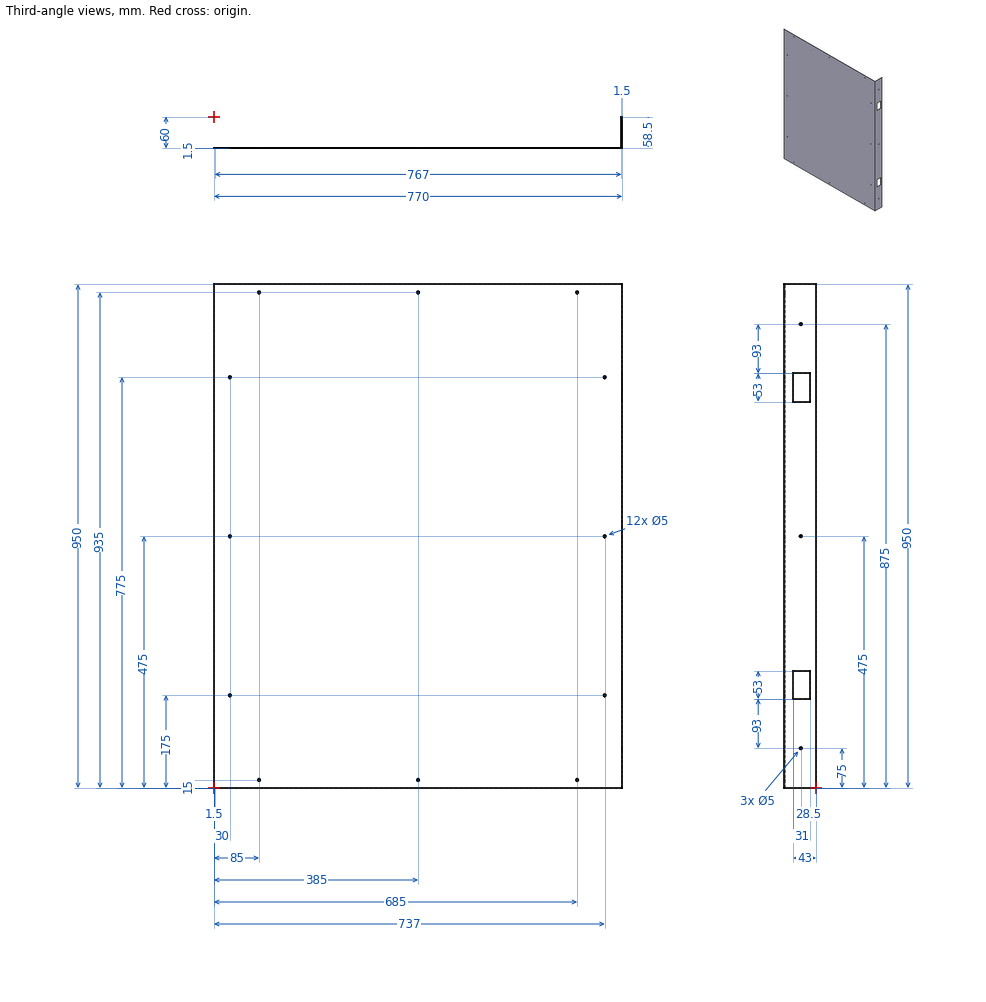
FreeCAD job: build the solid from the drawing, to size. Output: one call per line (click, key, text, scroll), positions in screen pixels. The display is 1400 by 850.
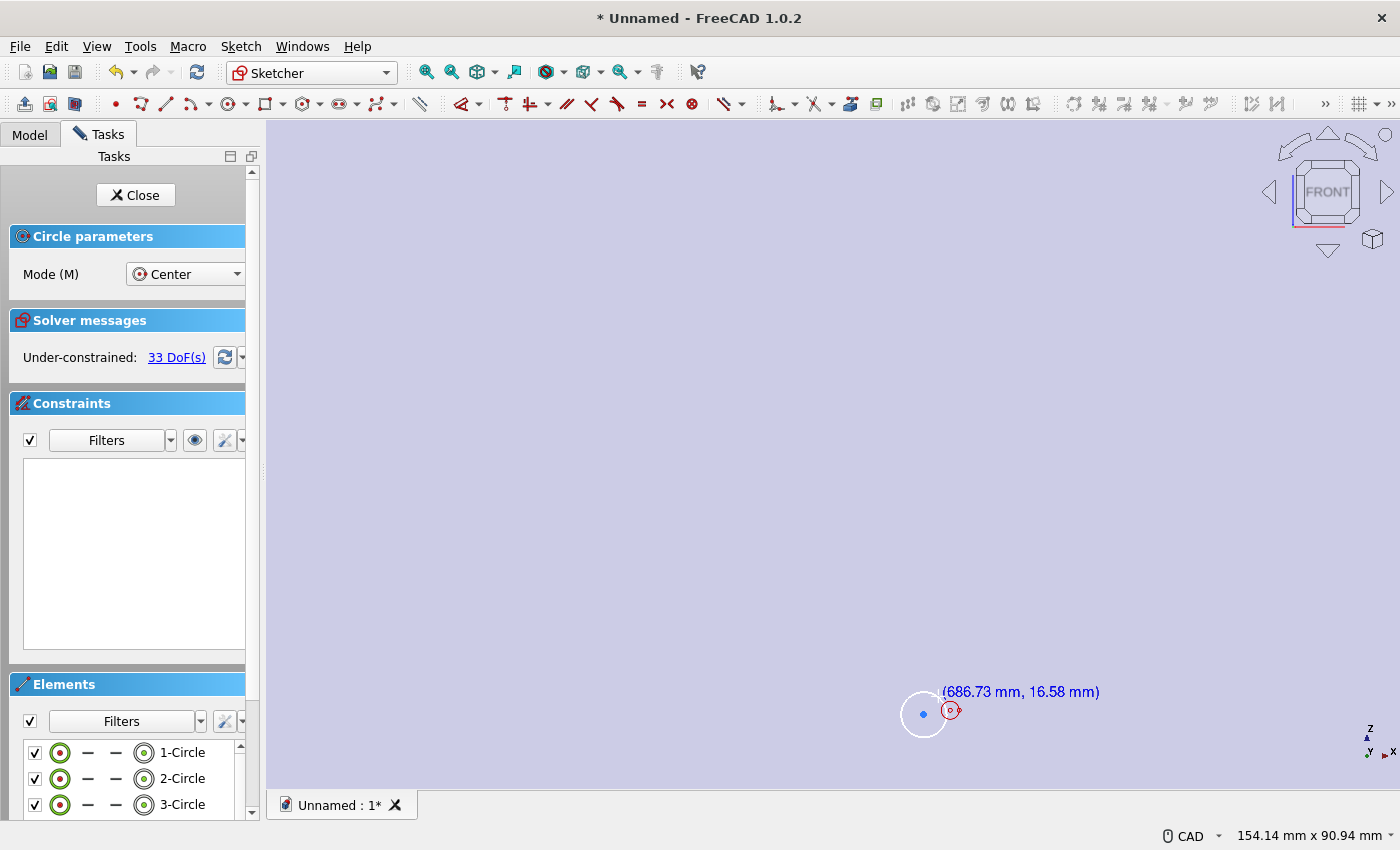
scroll(904, 654, down, 14)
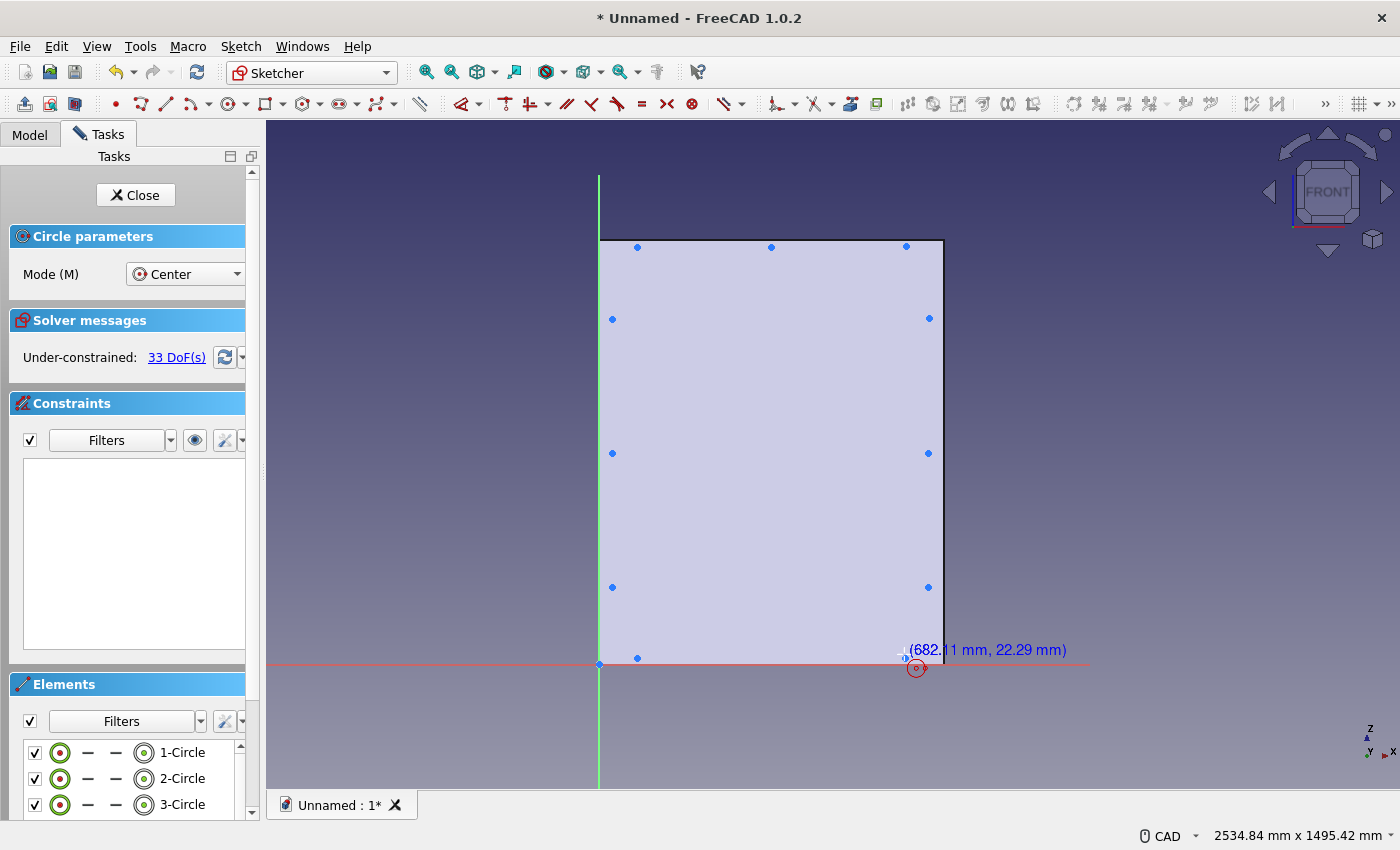
scroll(772, 658, up, 16)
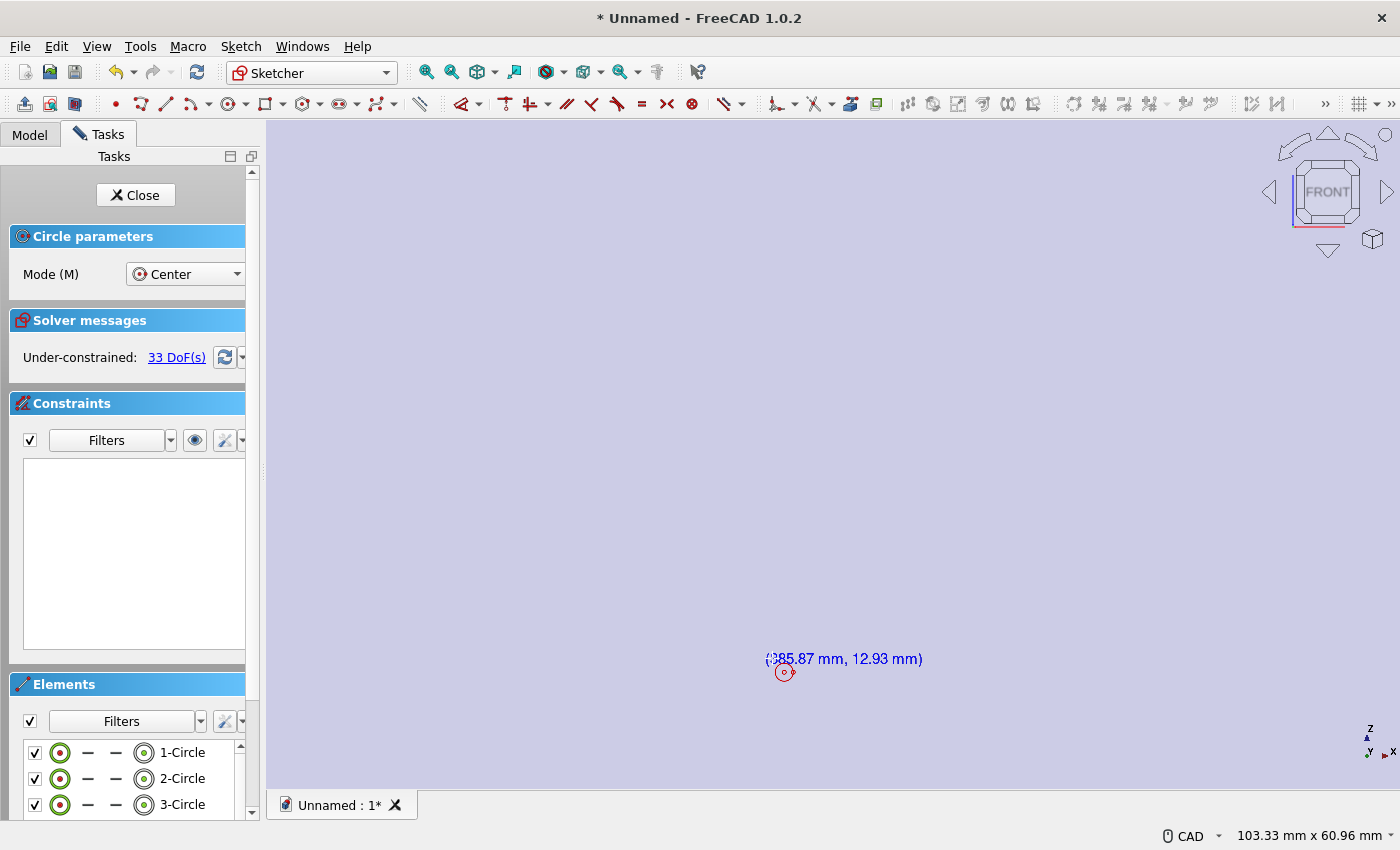
scroll(774, 706, down, 15)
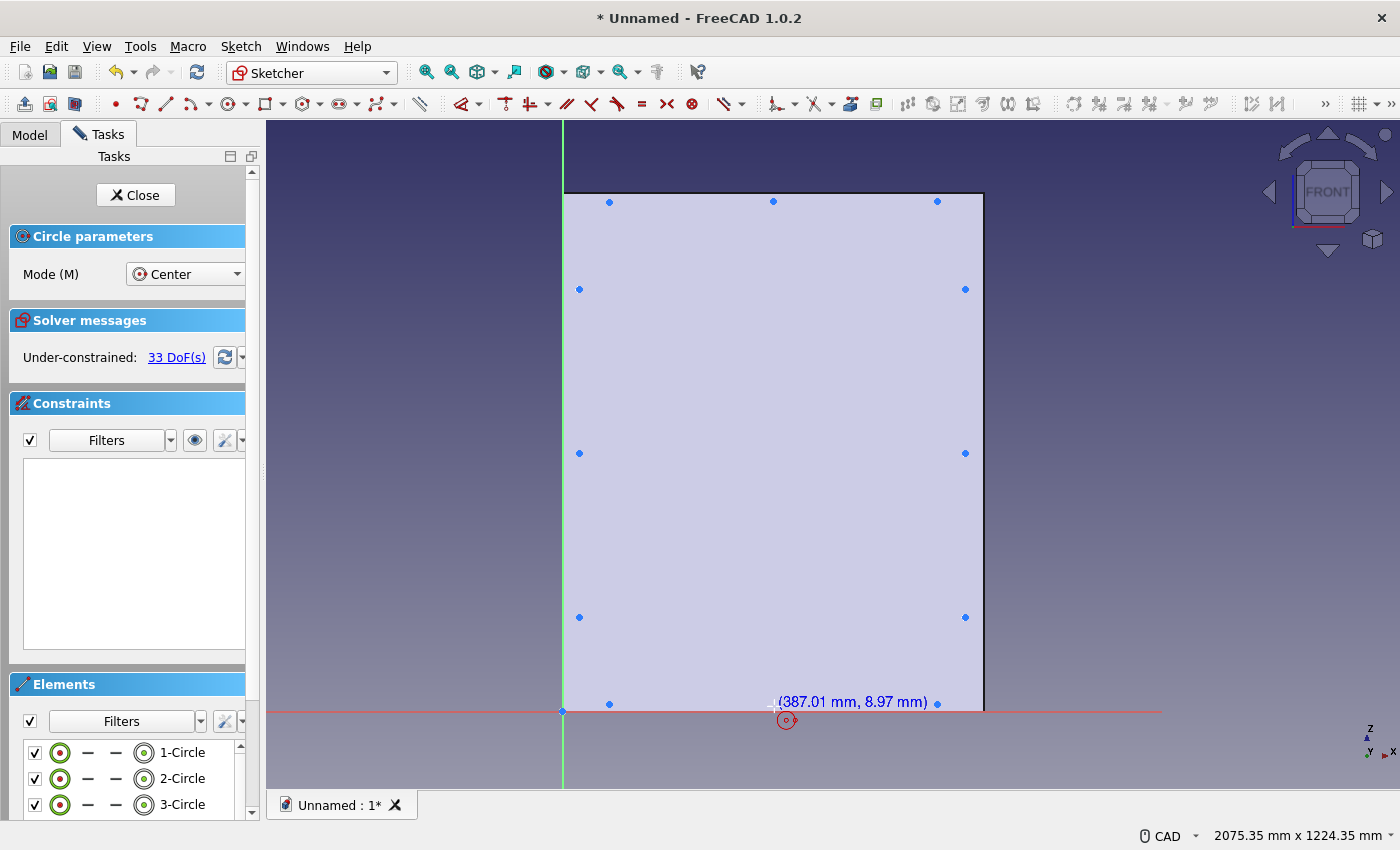
scroll(773, 704, up, 4)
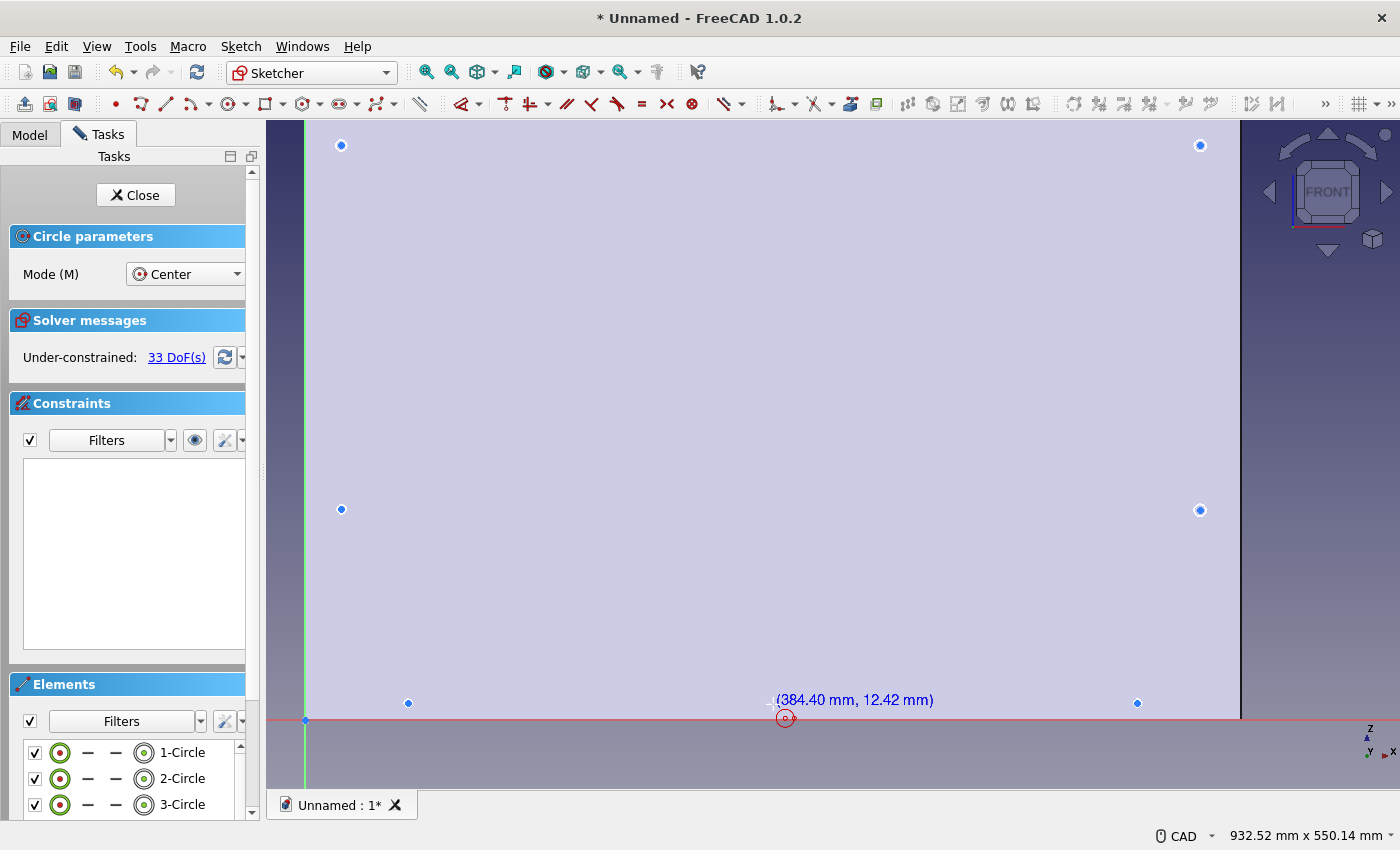
click(773, 702)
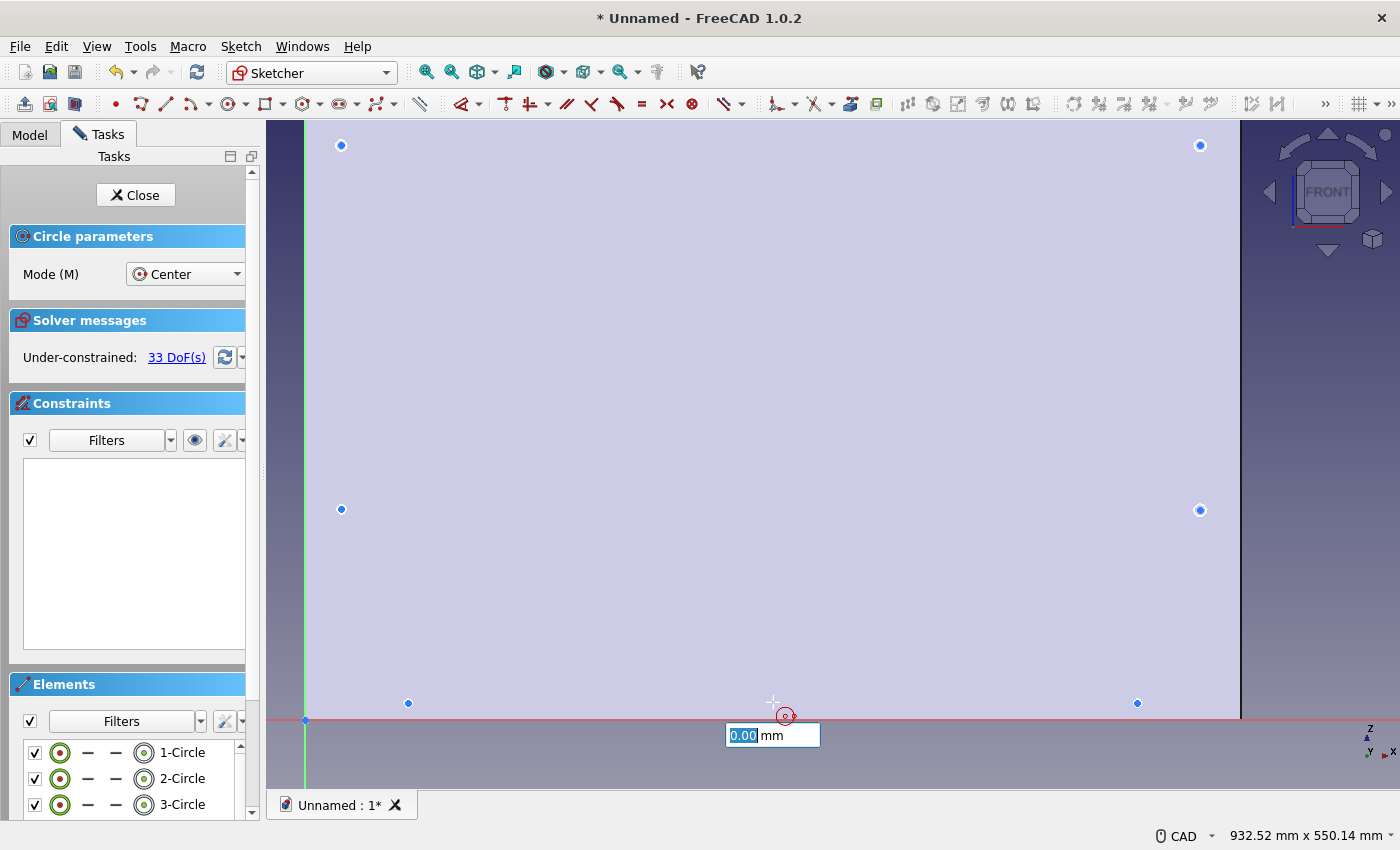
scroll(775, 700, up, 9)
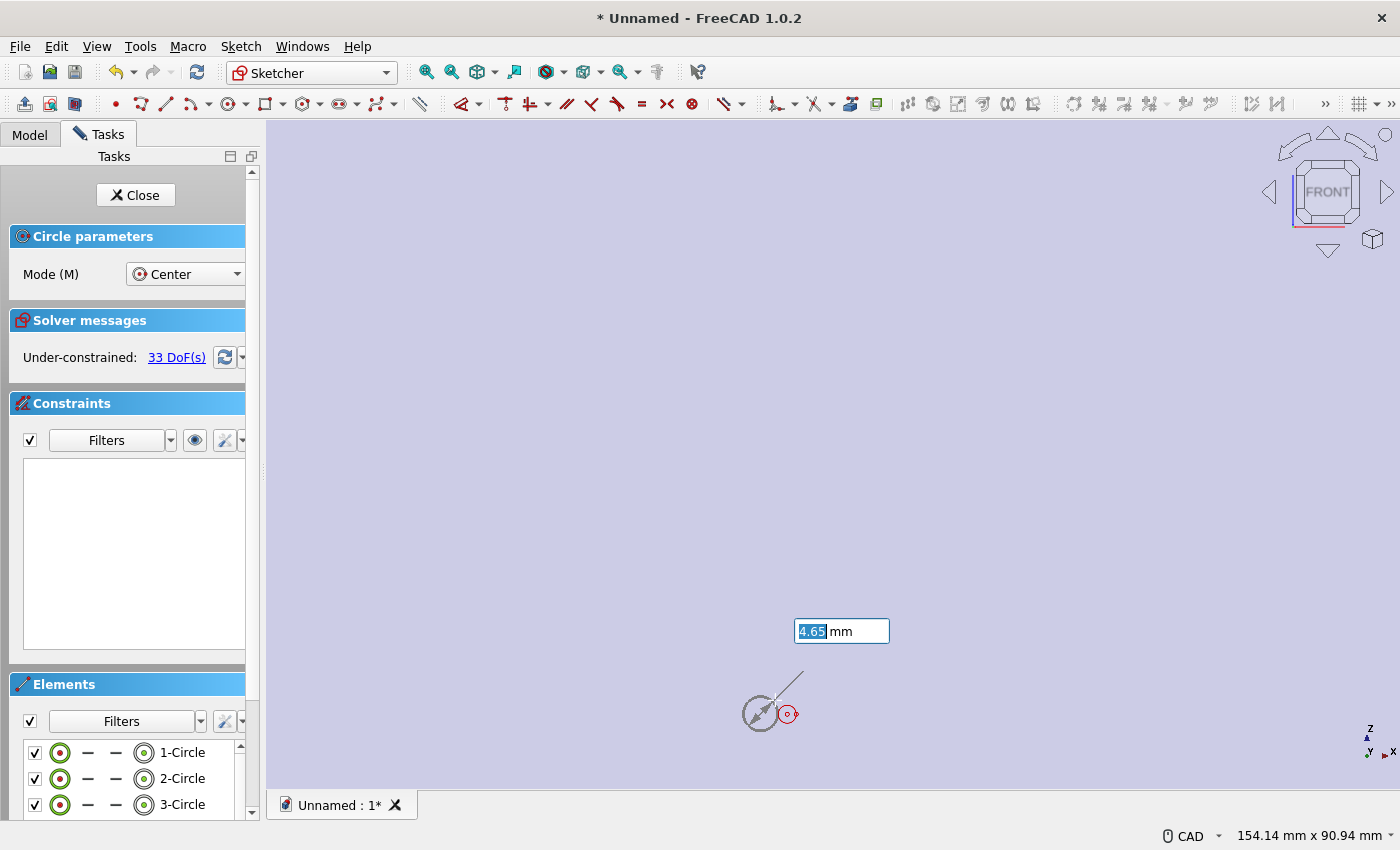
click(775, 695)
key(Escape)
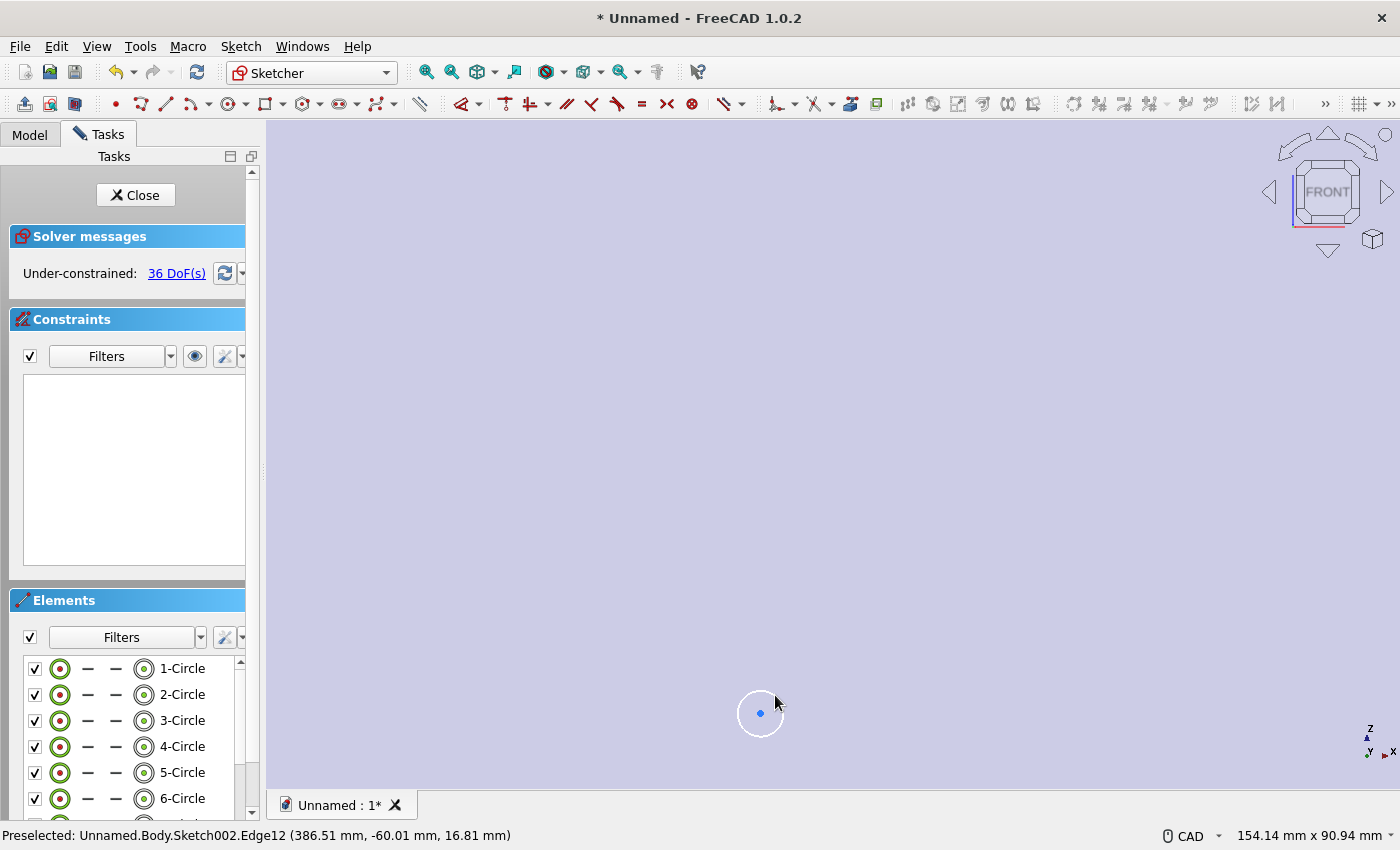
scroll(772, 654, down, 14)